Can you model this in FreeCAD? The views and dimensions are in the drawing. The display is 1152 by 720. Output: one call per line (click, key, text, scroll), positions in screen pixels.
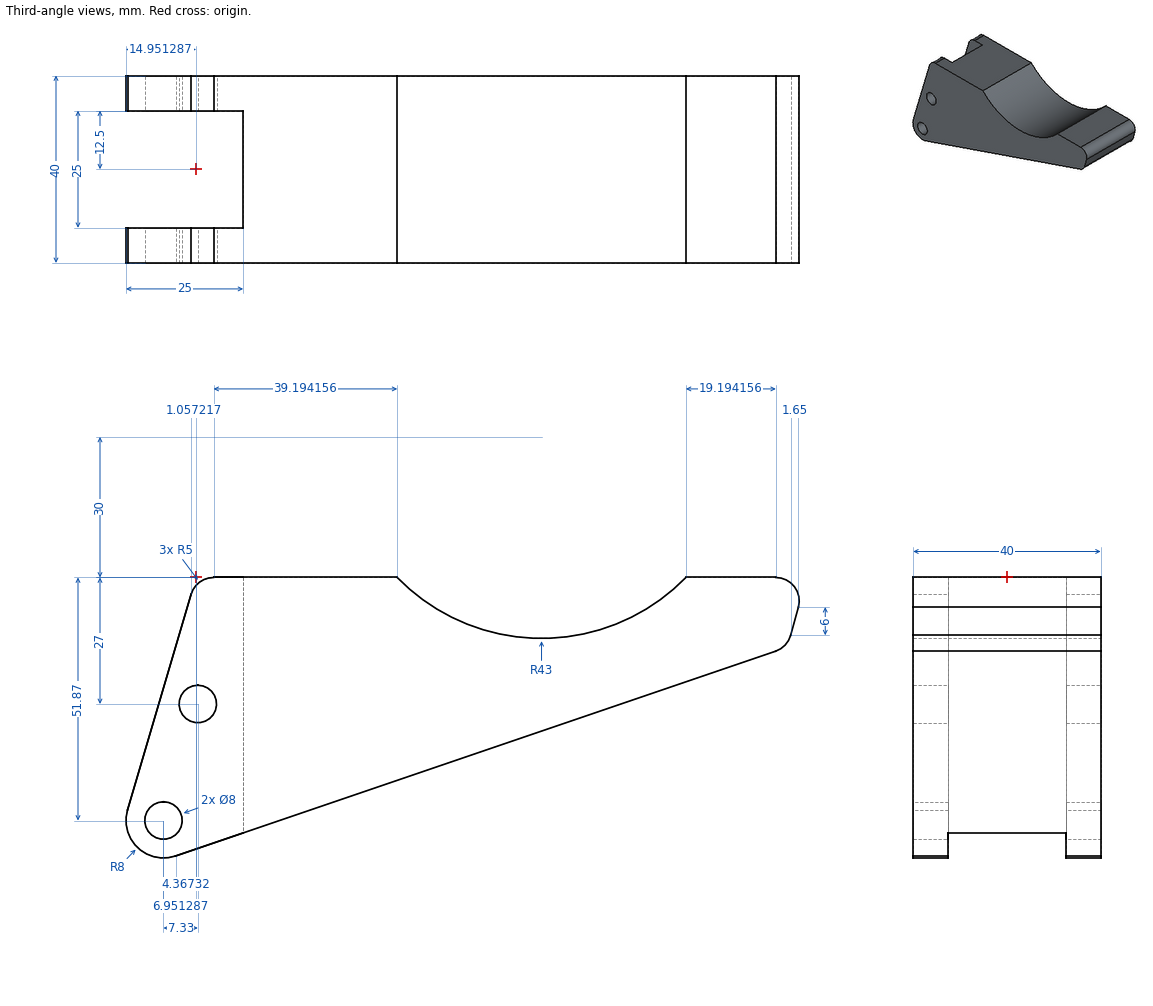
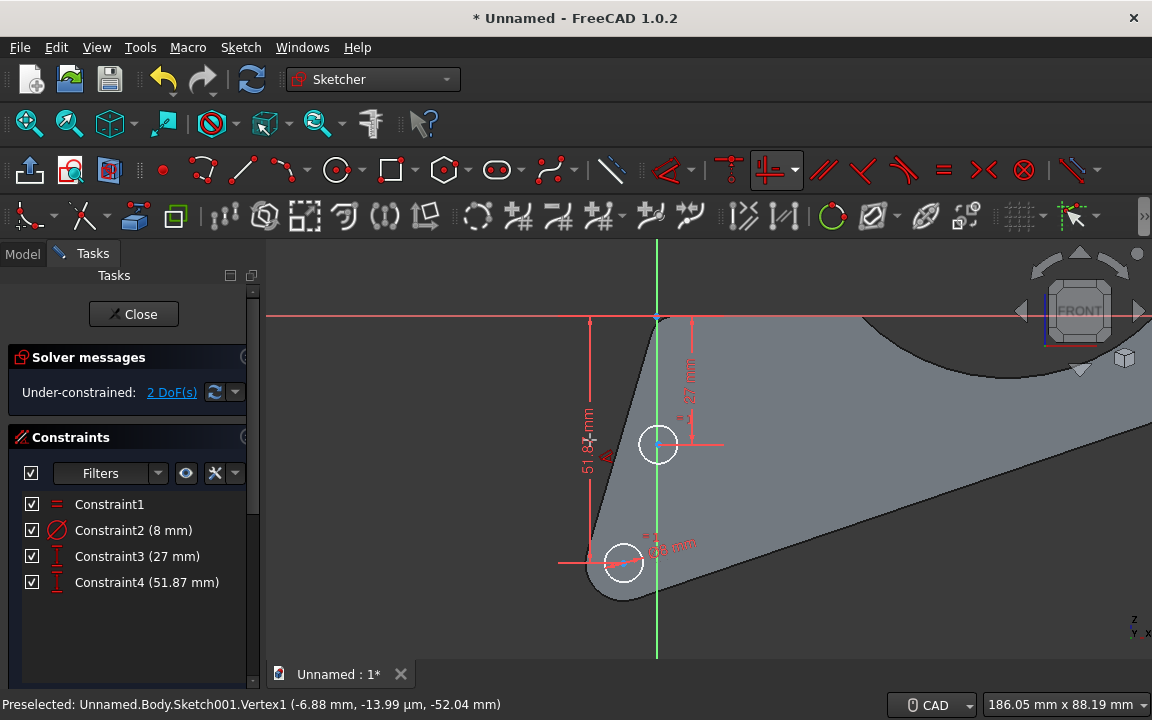
click(624, 563)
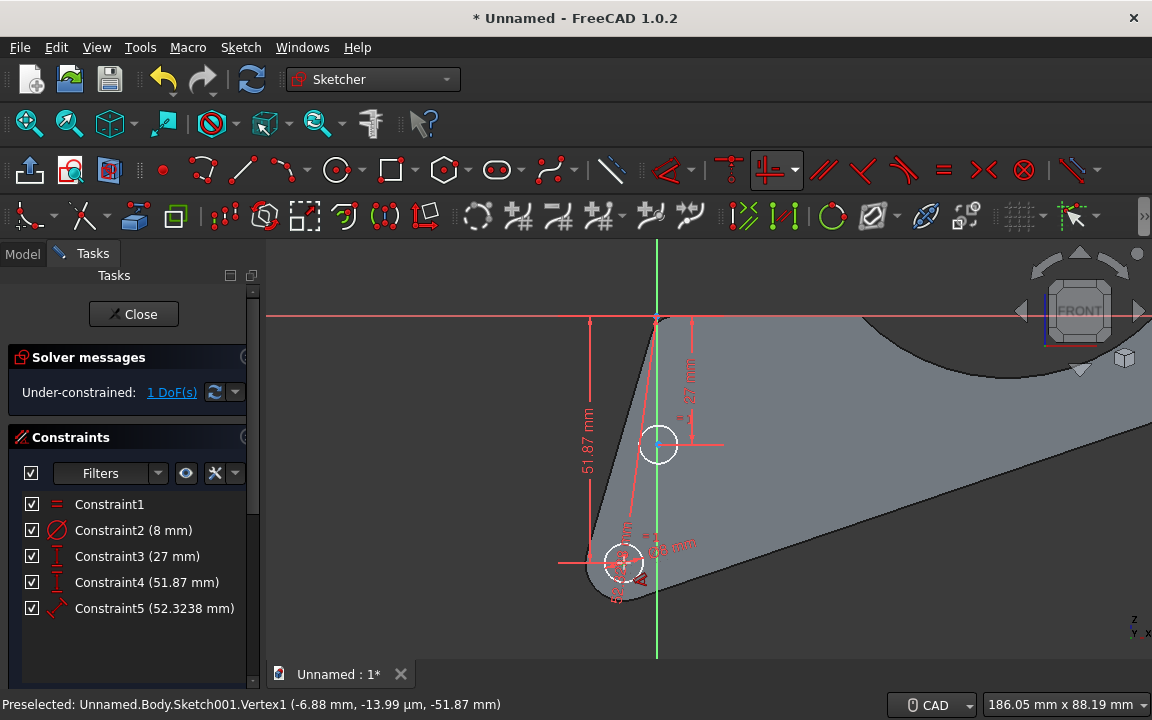
click(658, 445)
click(641, 597)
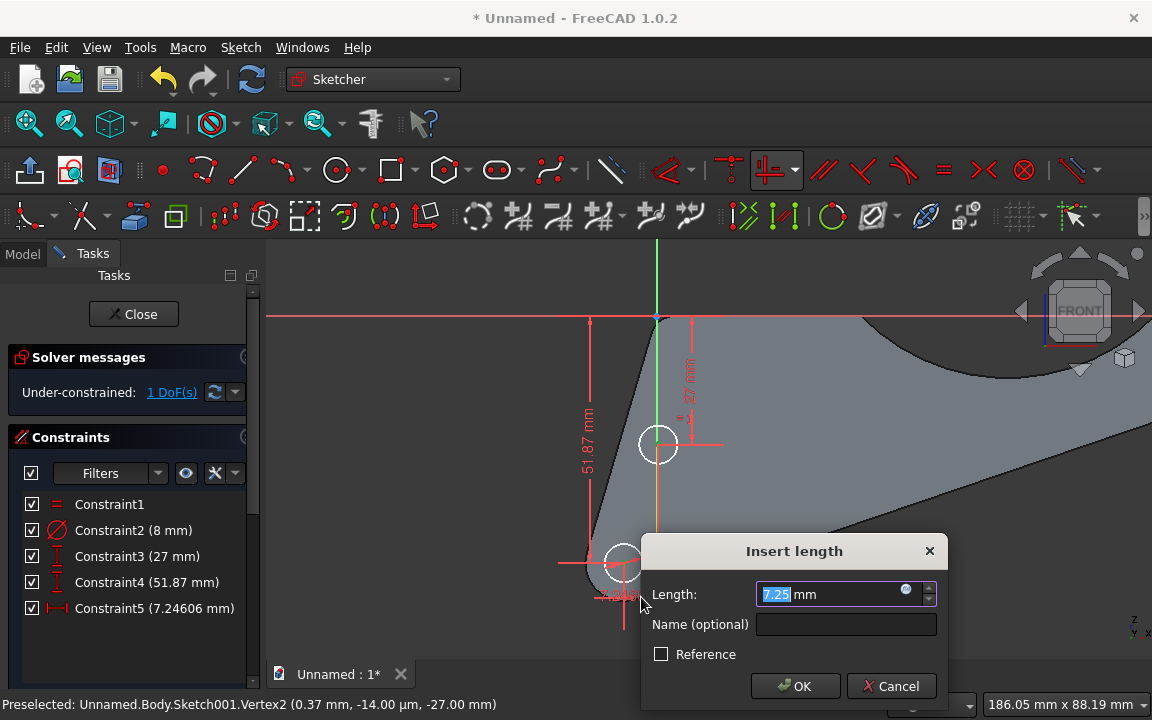
text(7.33)
key(Return)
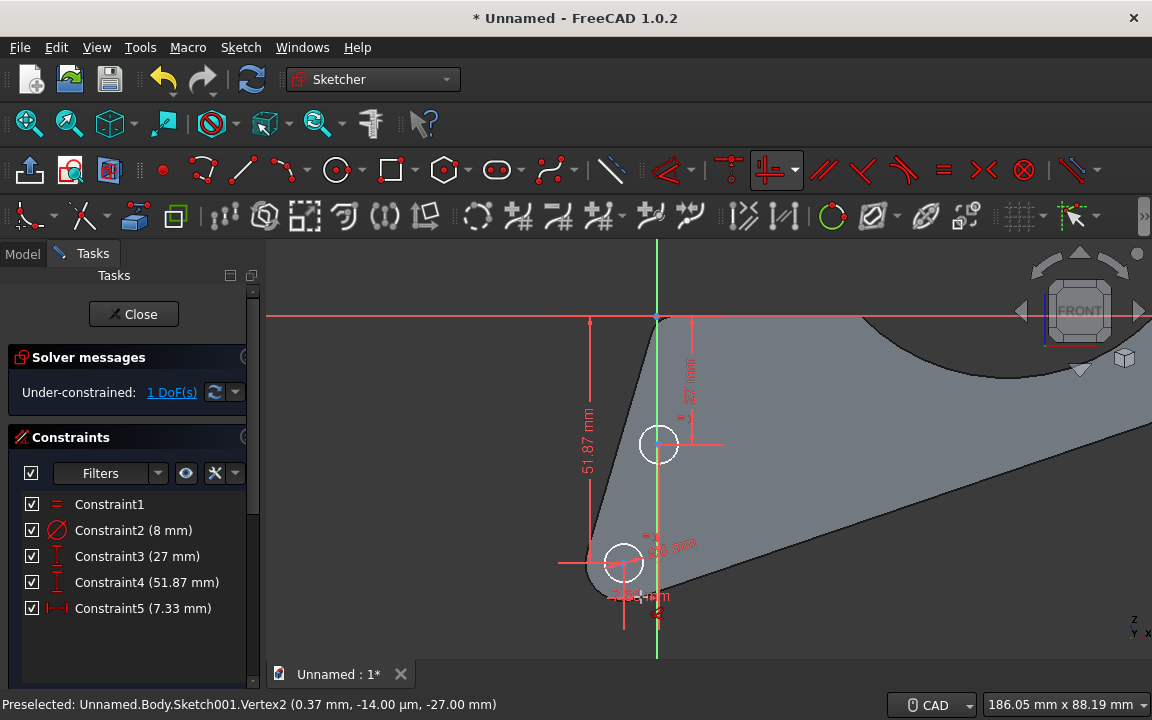
click(624, 563)
click(640, 282)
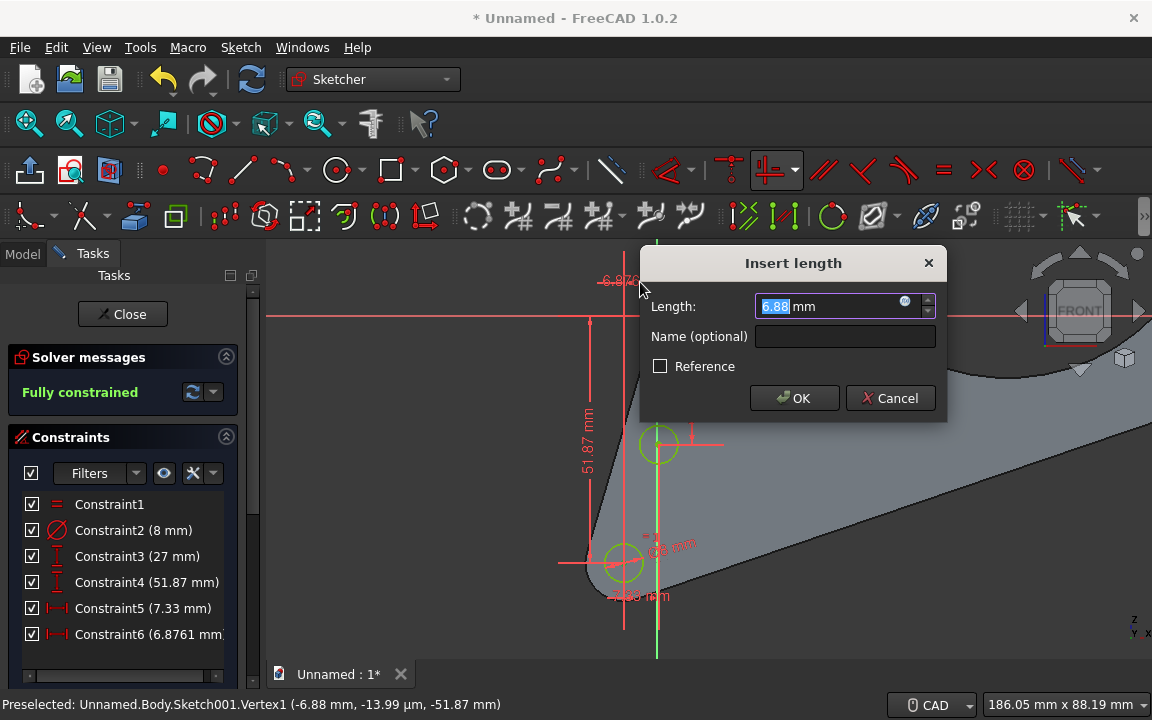
text(6.951287)
key(Return)
key(Escape)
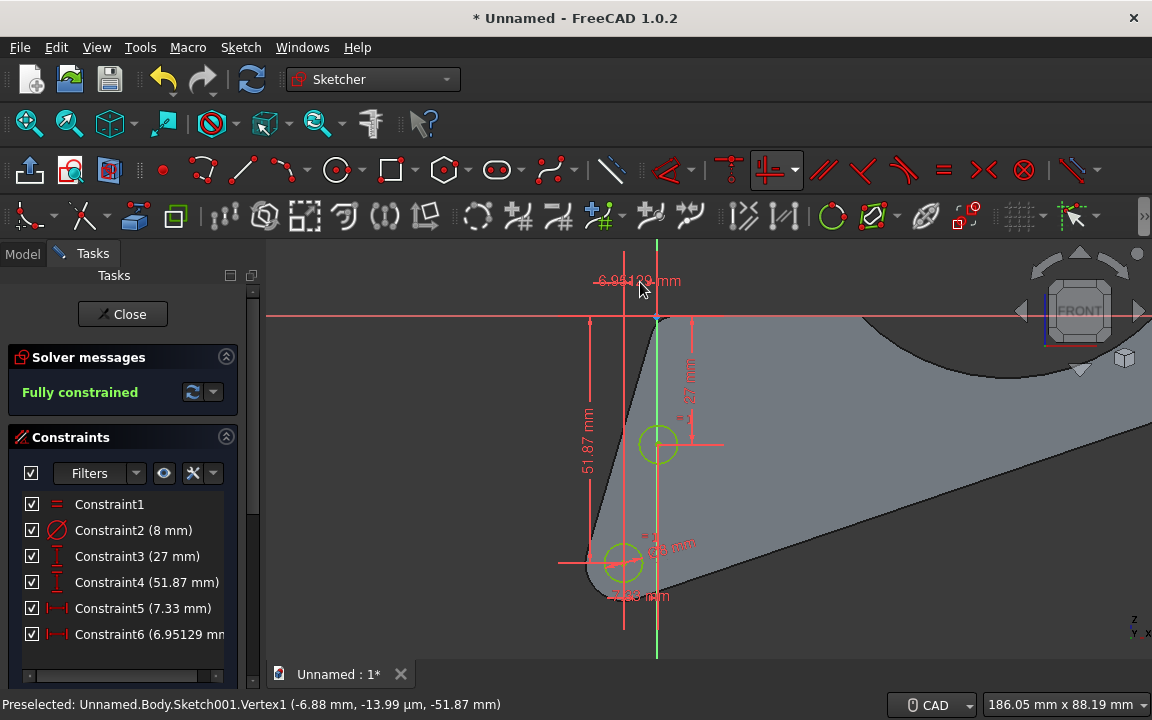
click(123, 314)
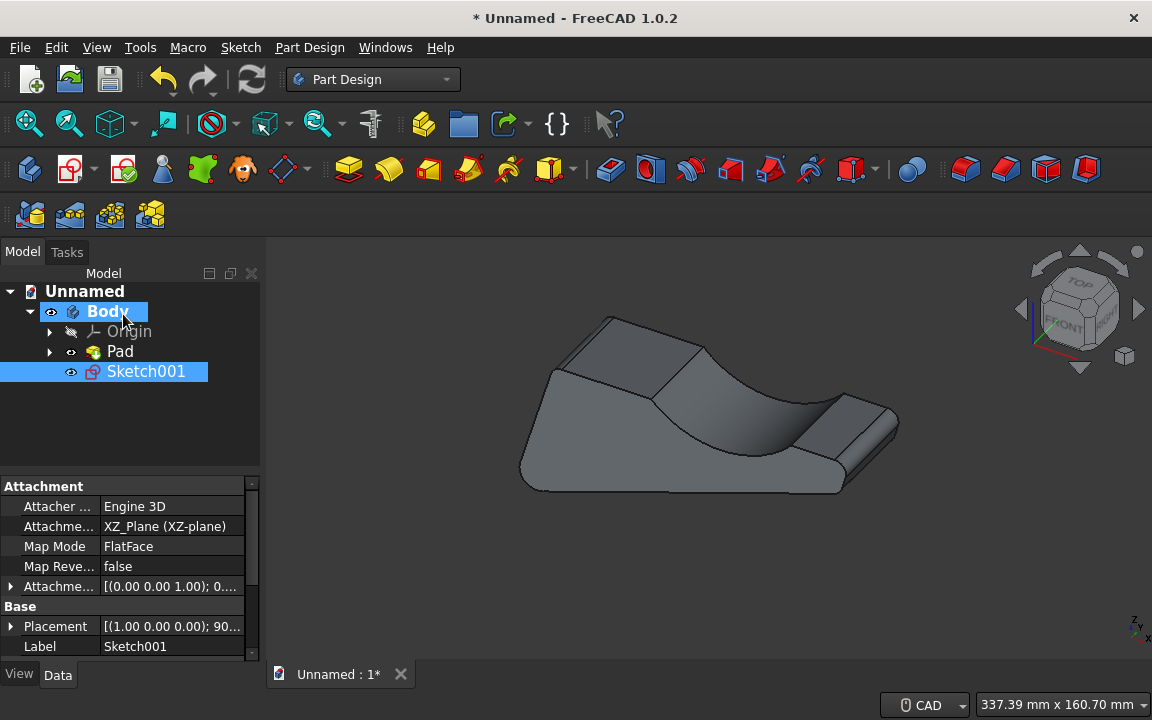
click(612, 170)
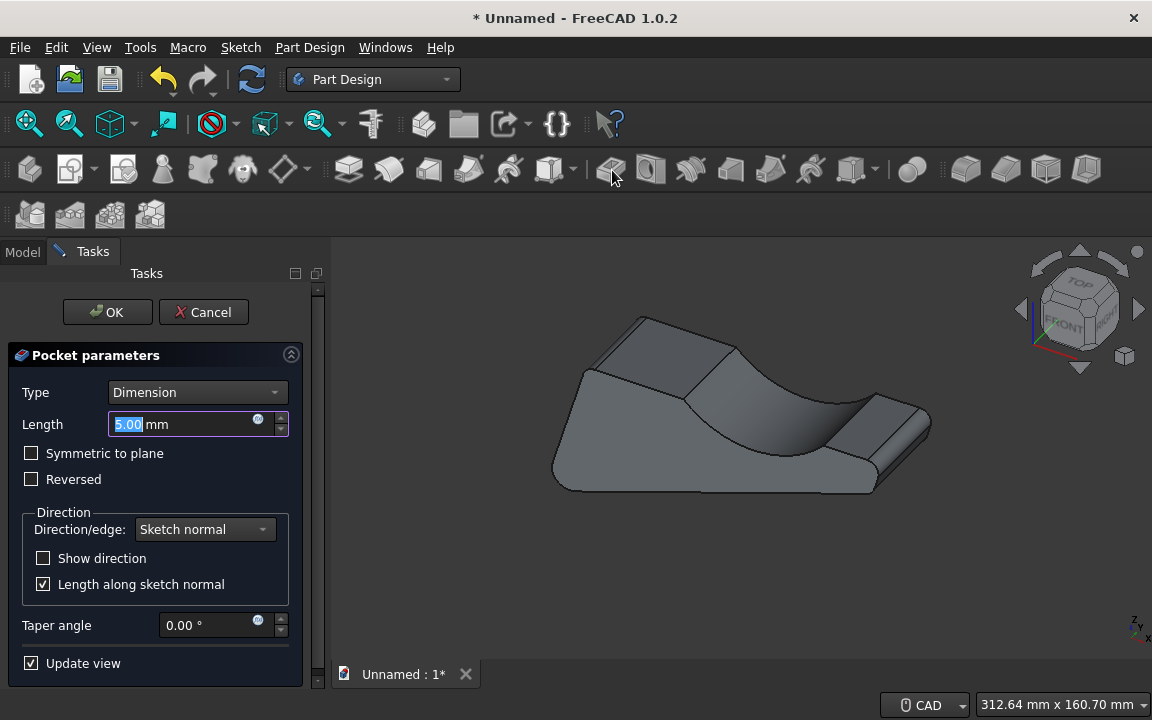
text(40)
key(Tab)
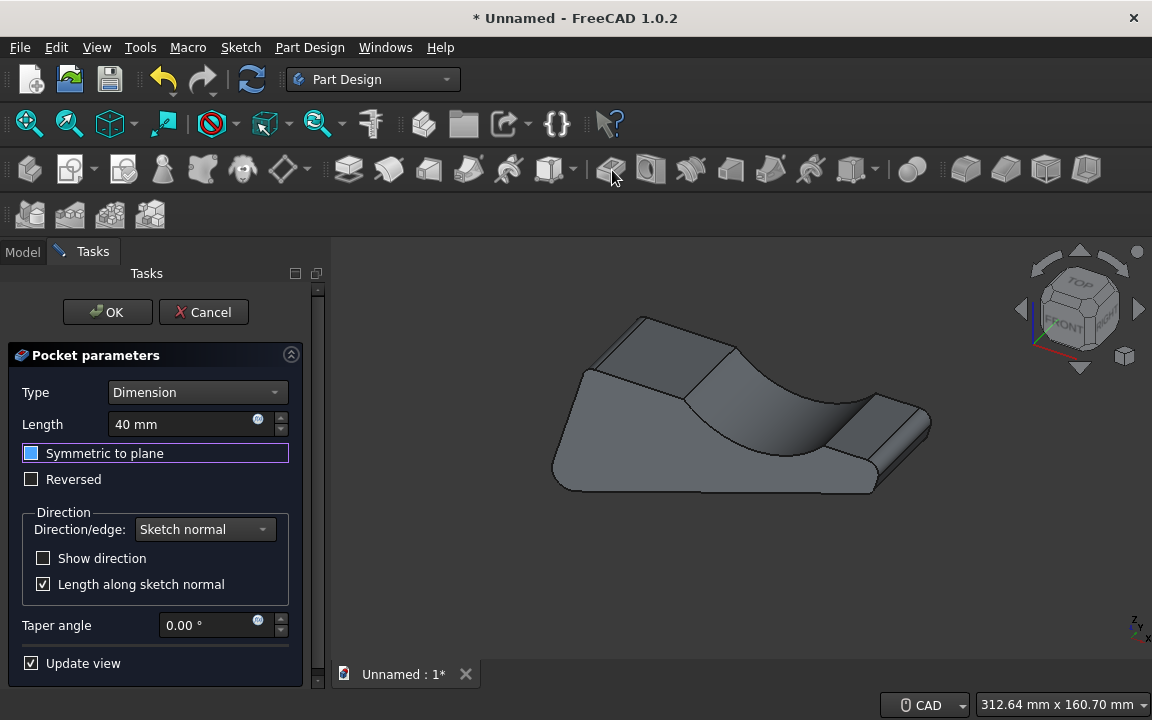
click(30, 453)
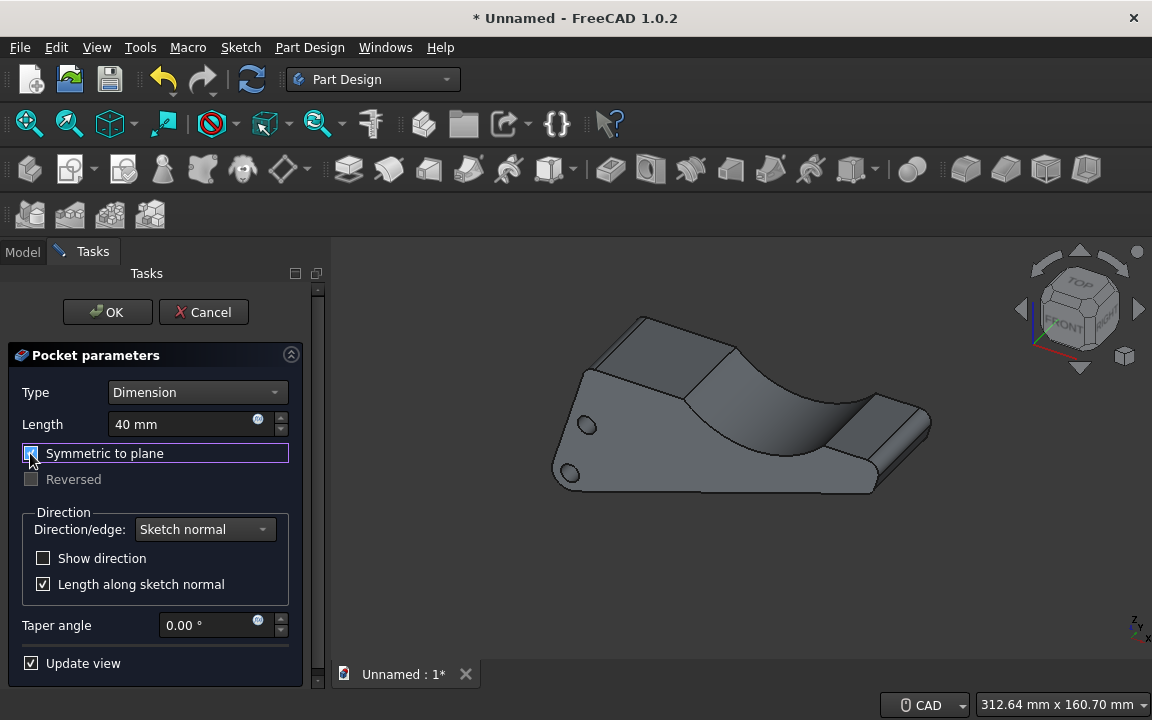
click(108, 312)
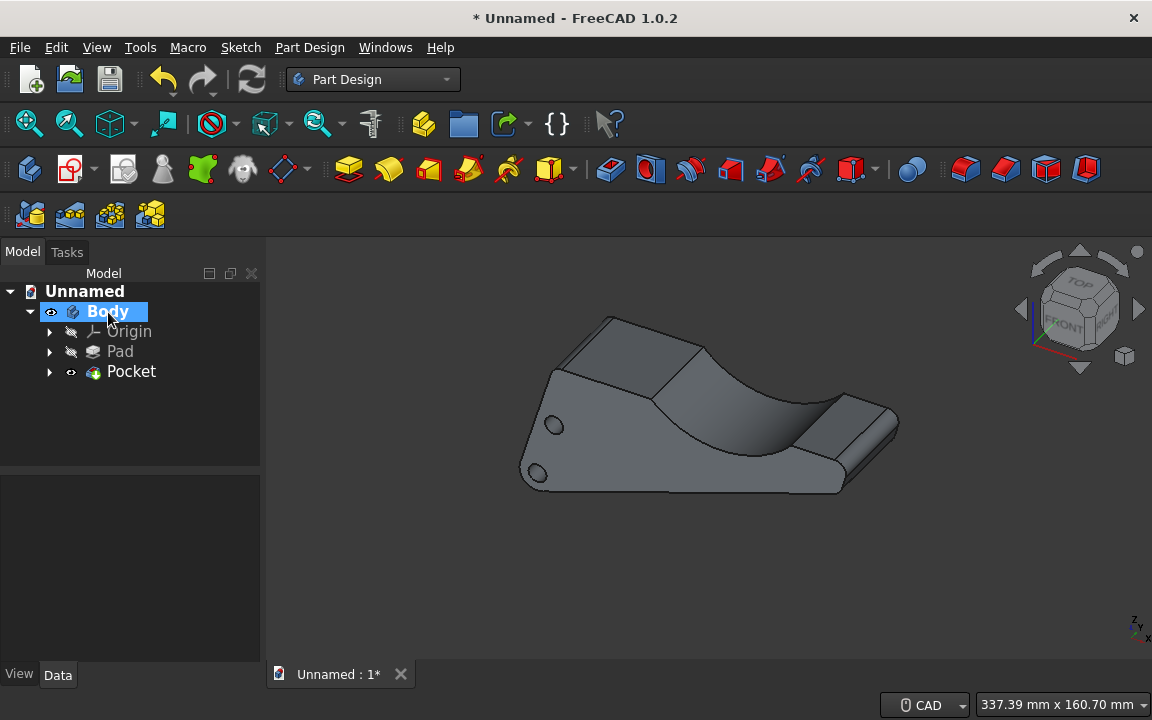
click(70, 170)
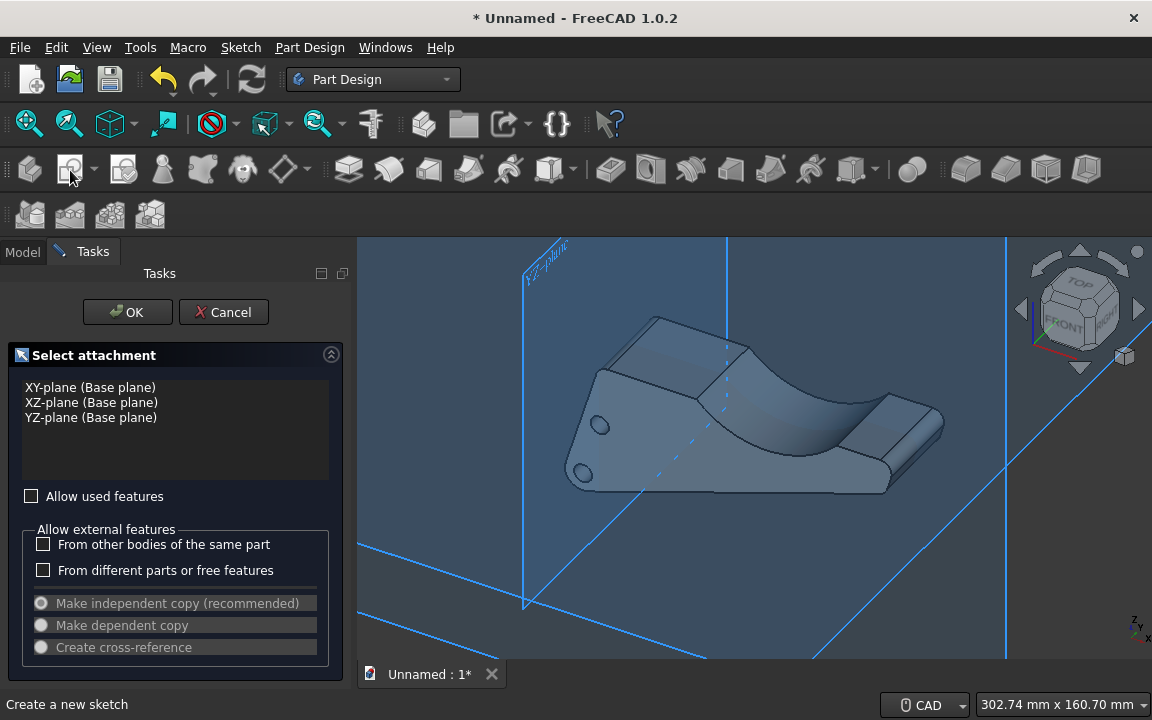
click(82, 388)